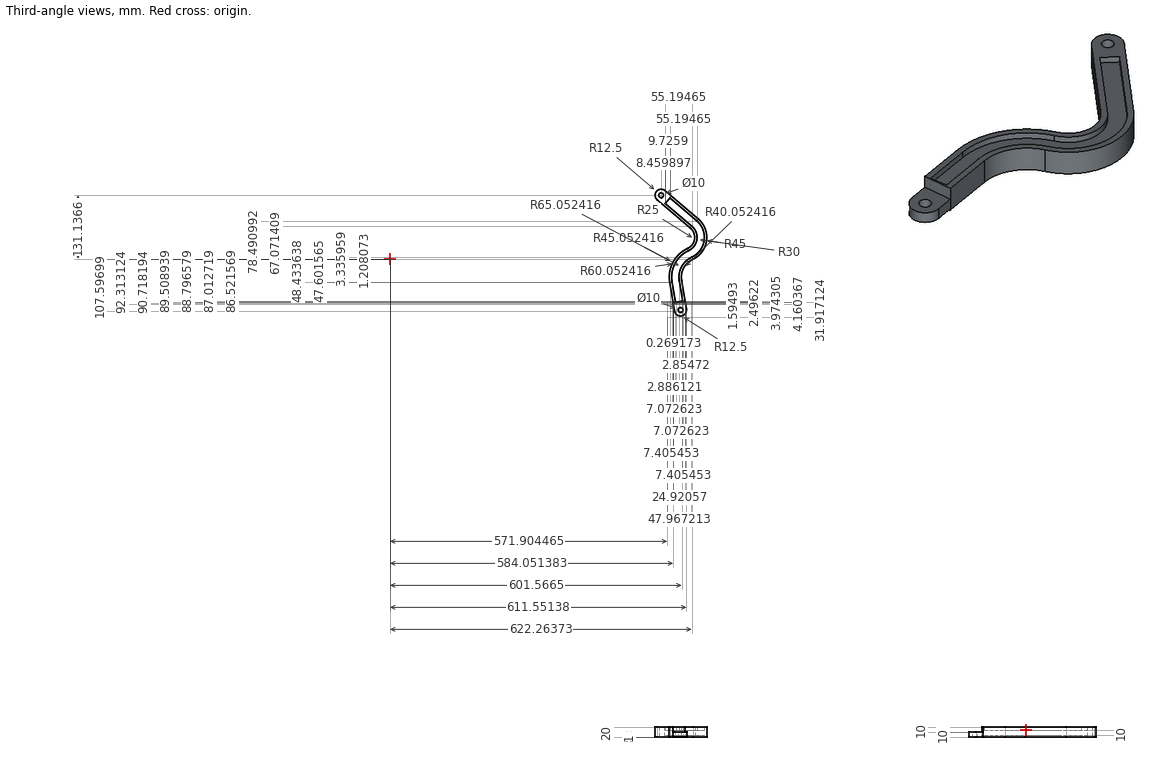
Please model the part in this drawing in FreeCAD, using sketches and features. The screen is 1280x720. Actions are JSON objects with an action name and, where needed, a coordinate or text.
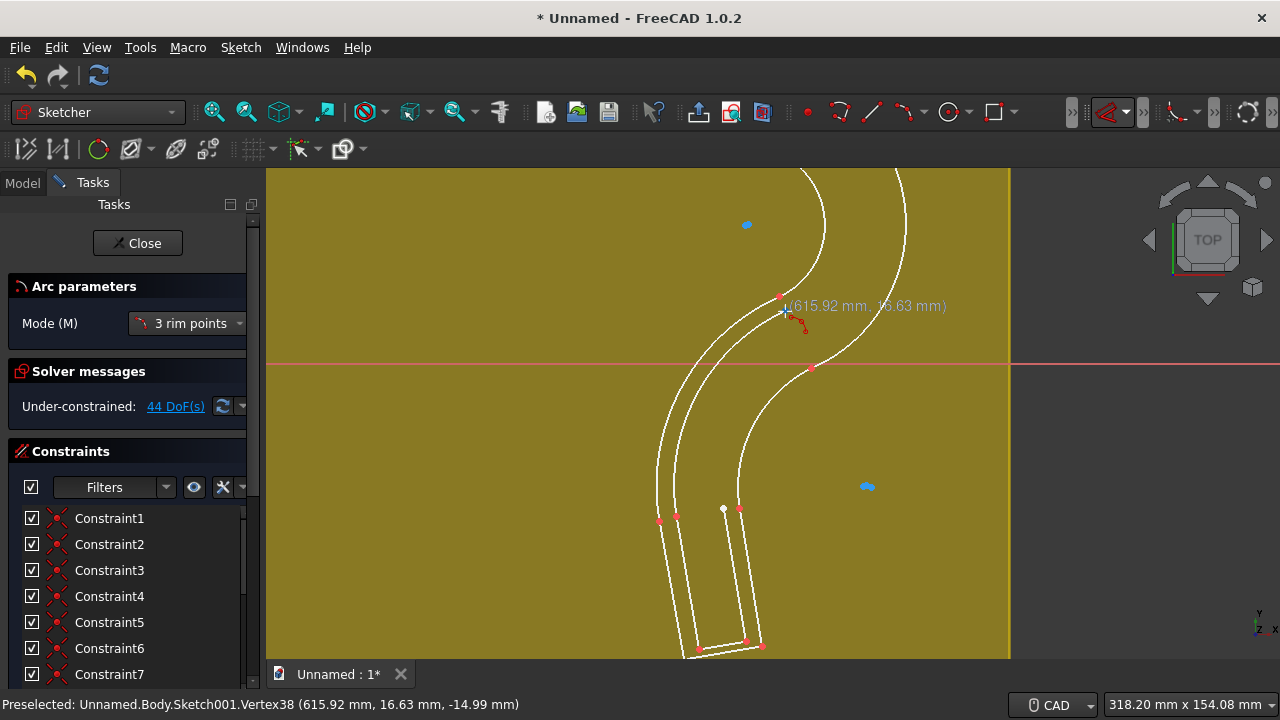
{"action": "scroll", "coordinate": [677, 517], "scroll_direction": "down", "scroll_amount": 4}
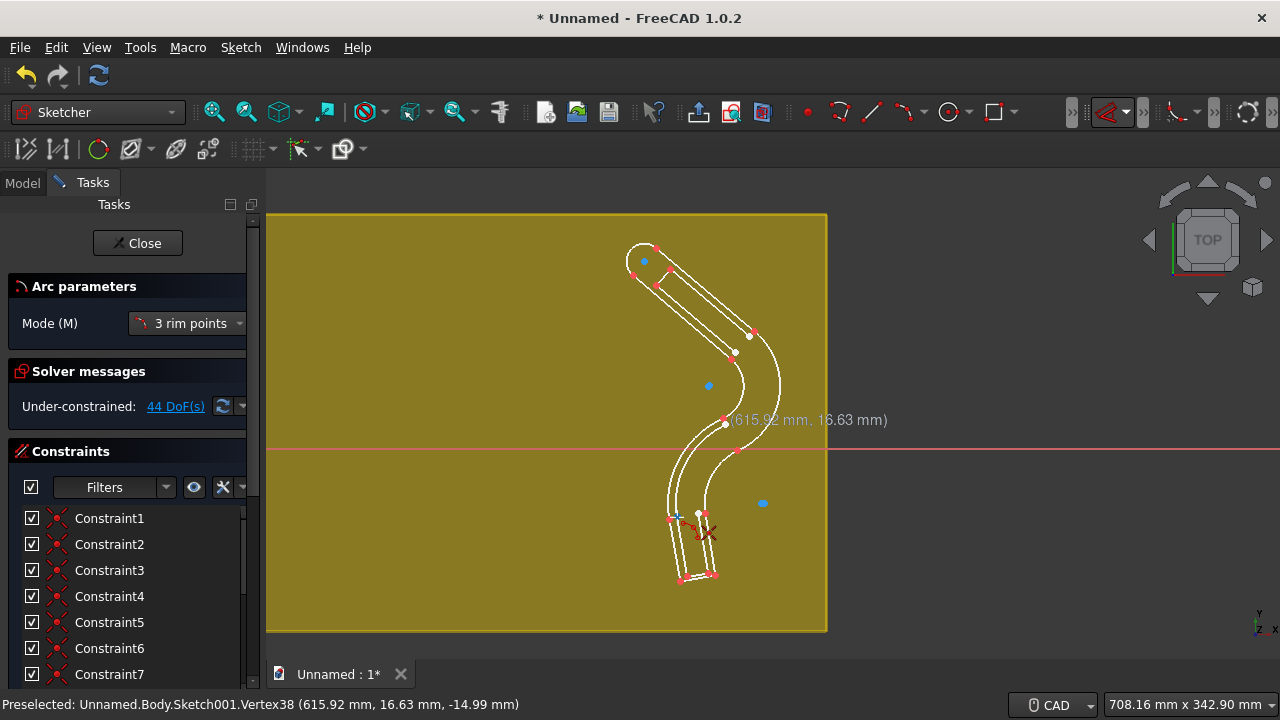
{"action": "scroll", "coordinate": [736, 353], "scroll_direction": "up", "scroll_amount": 4}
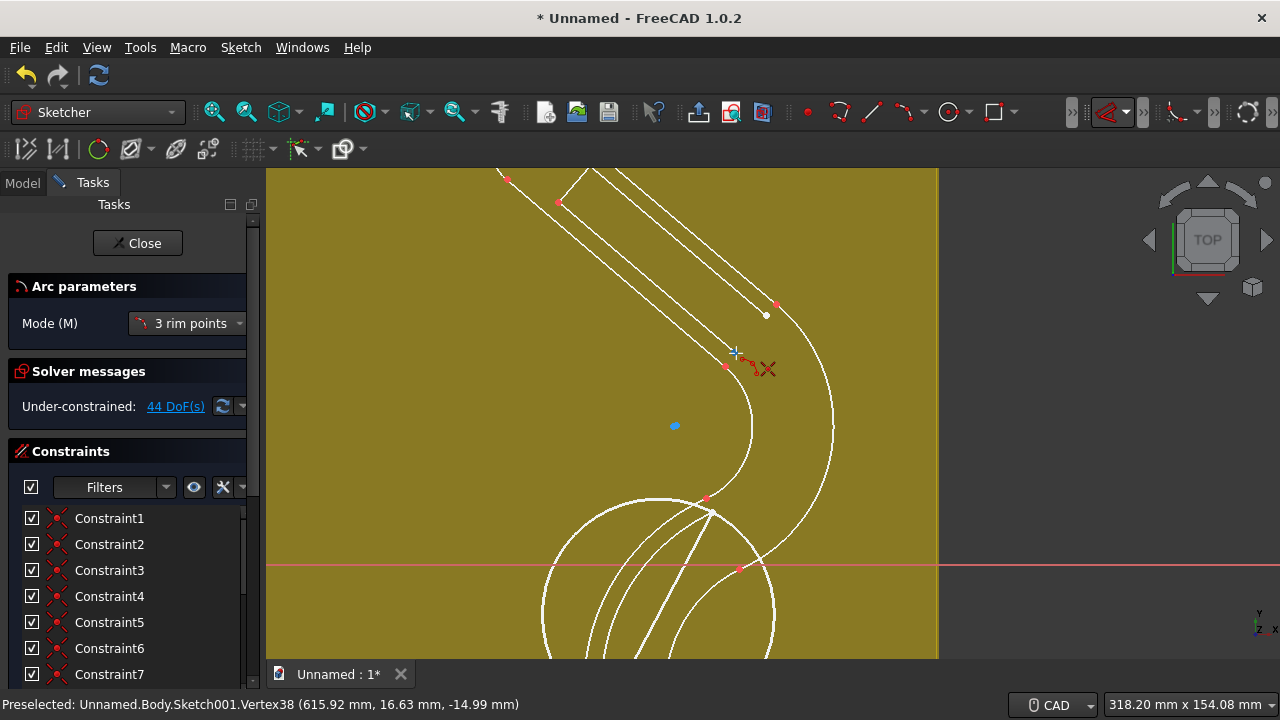
{"action": "left_click", "coordinate": [735, 352]}
{"action": "left_click", "coordinate": [768, 418]}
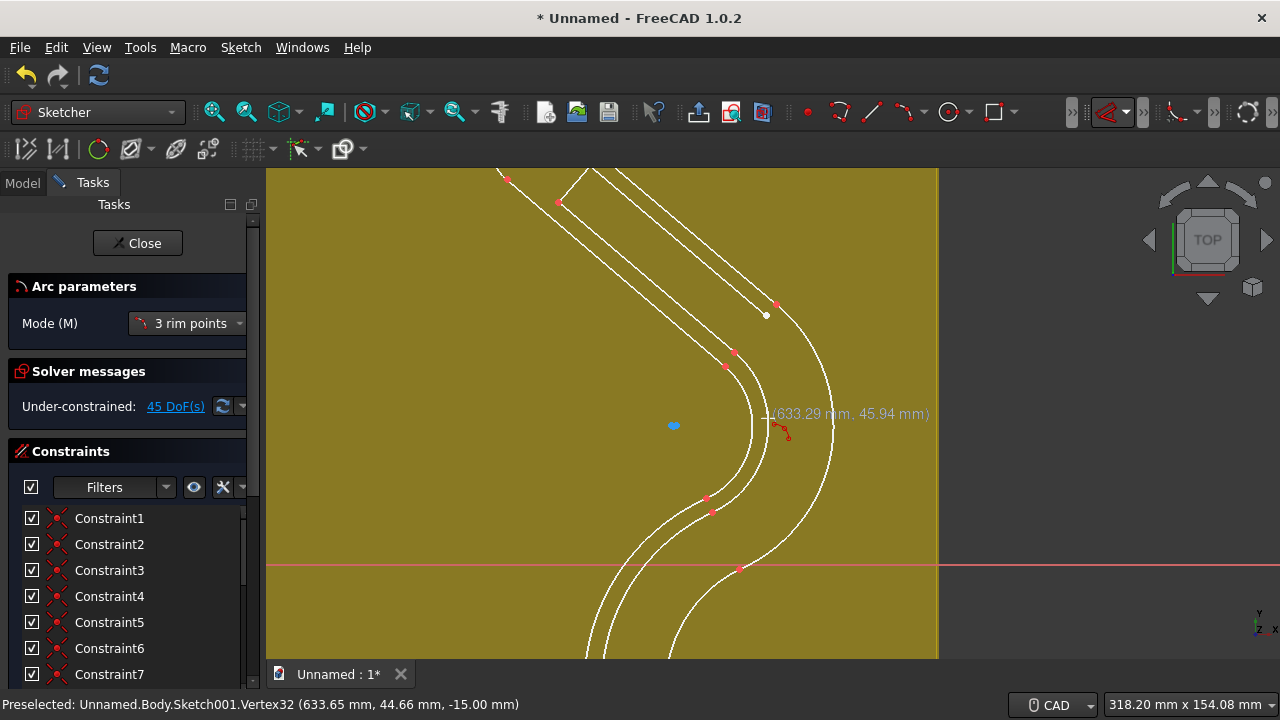
{"action": "left_click", "coordinate": [766, 316]}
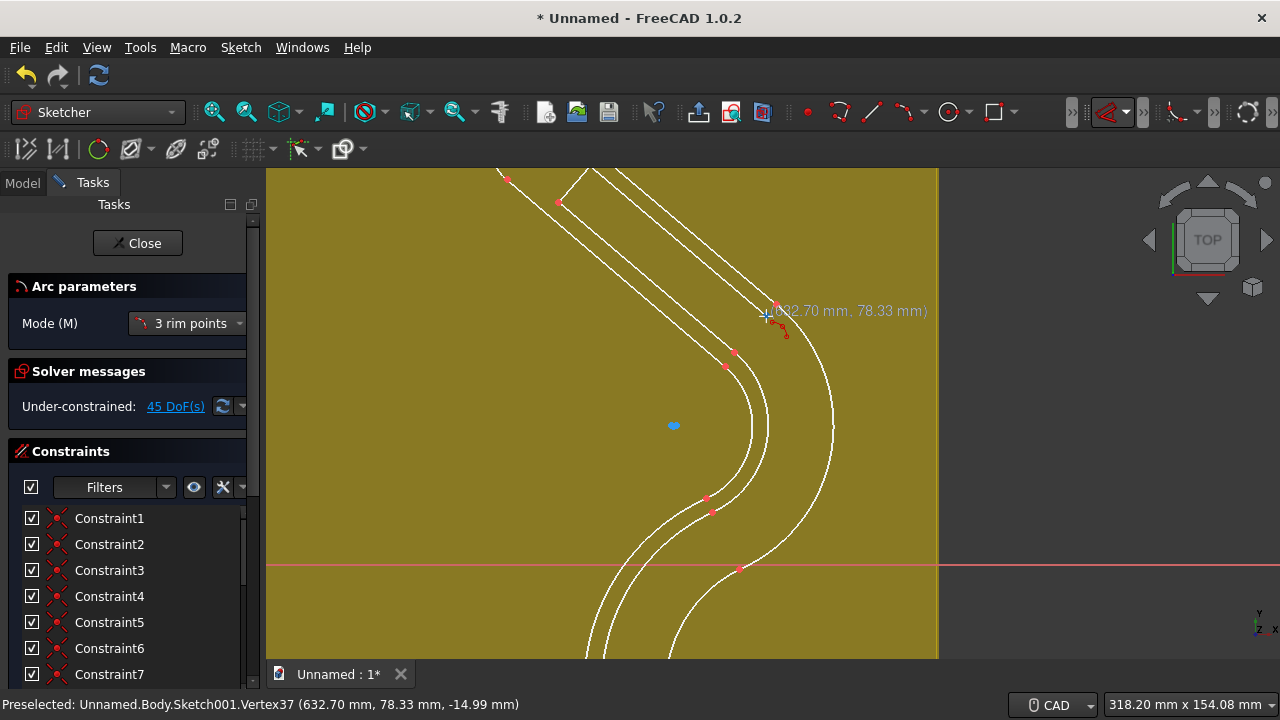
{"action": "scroll", "coordinate": [733, 555], "scroll_direction": "up", "scroll_amount": 3}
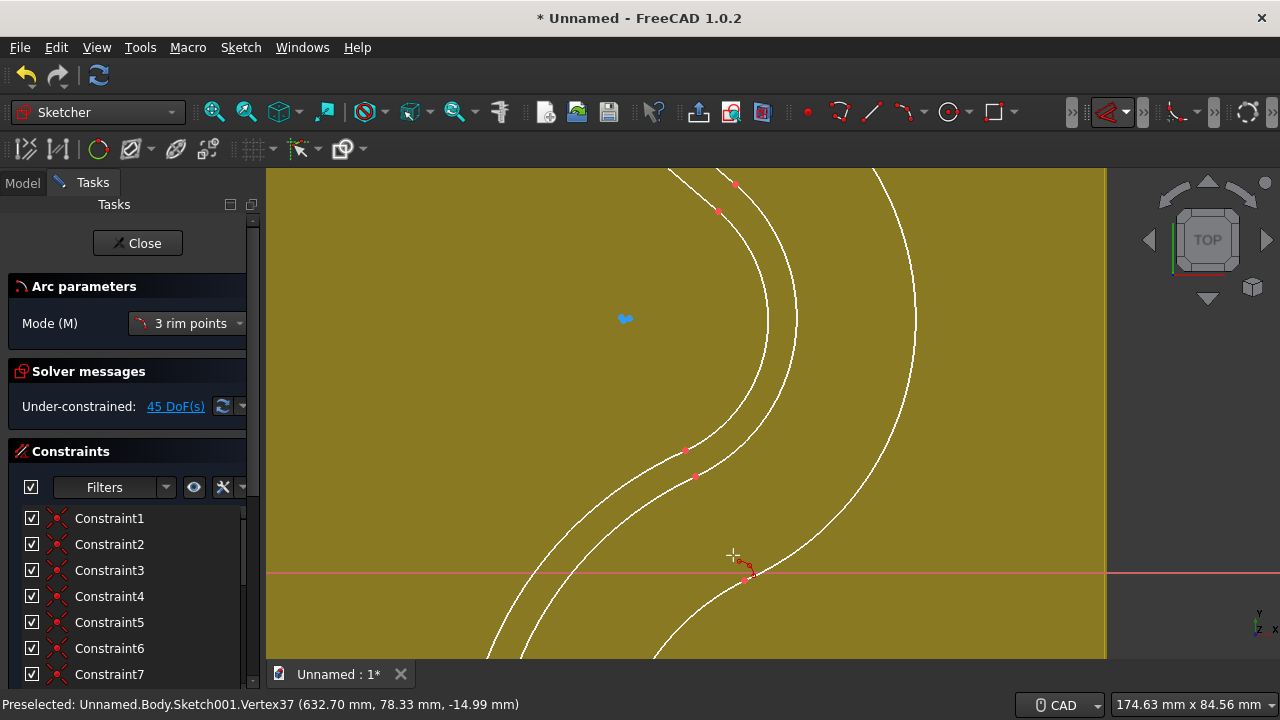
{"action": "left_click", "coordinate": [732, 554]}
{"action": "left_click", "coordinate": [884, 300]}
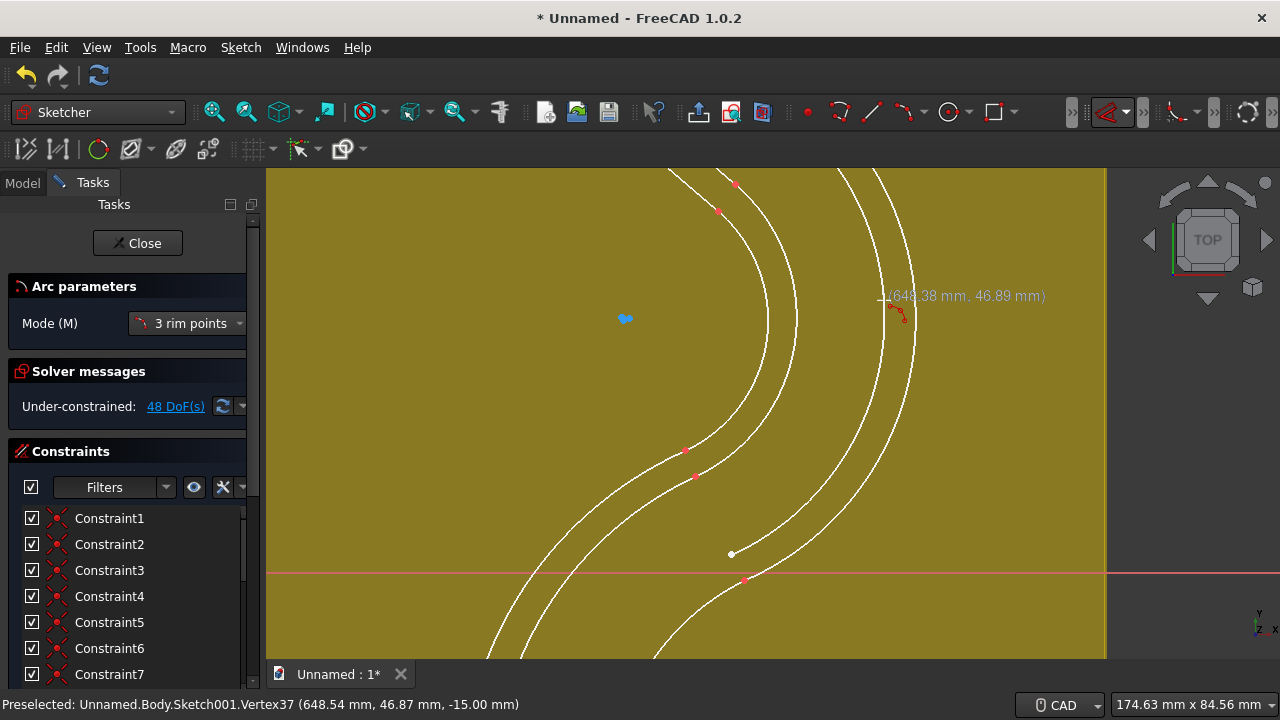
{"action": "left_click", "coordinate": [732, 555]}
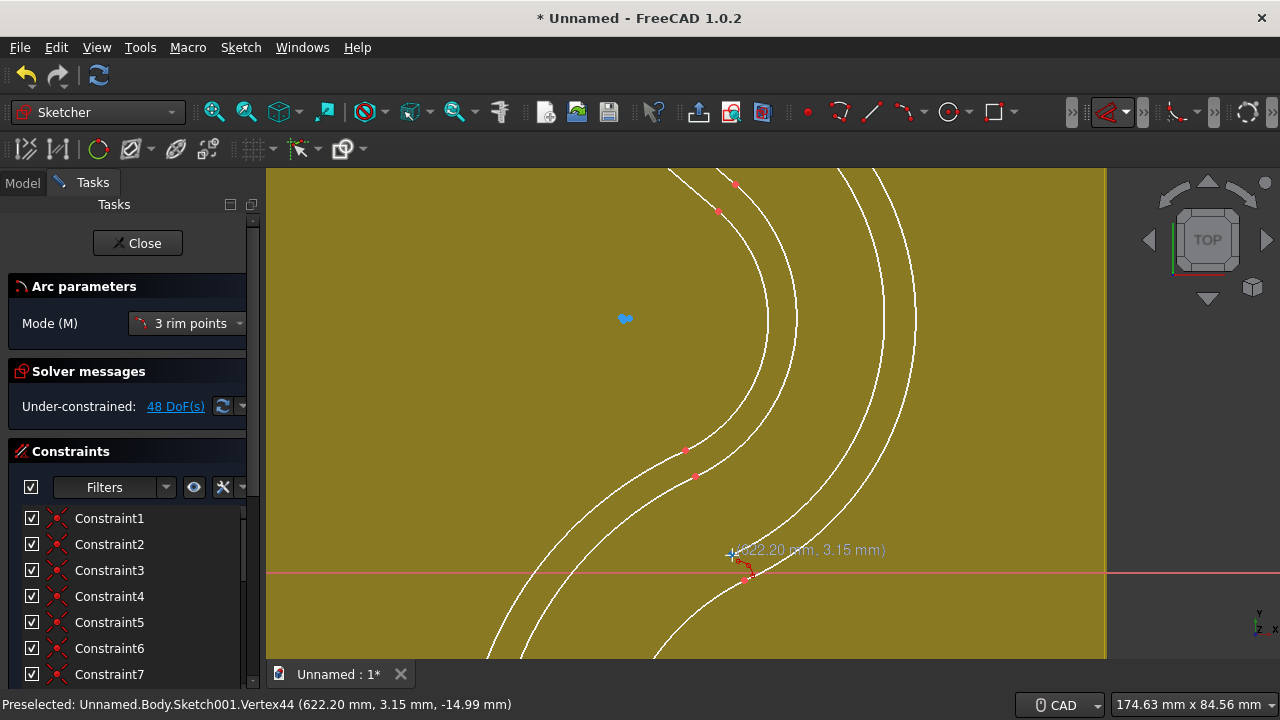
{"action": "scroll", "coordinate": [735, 407], "scroll_direction": "down", "scroll_amount": 7}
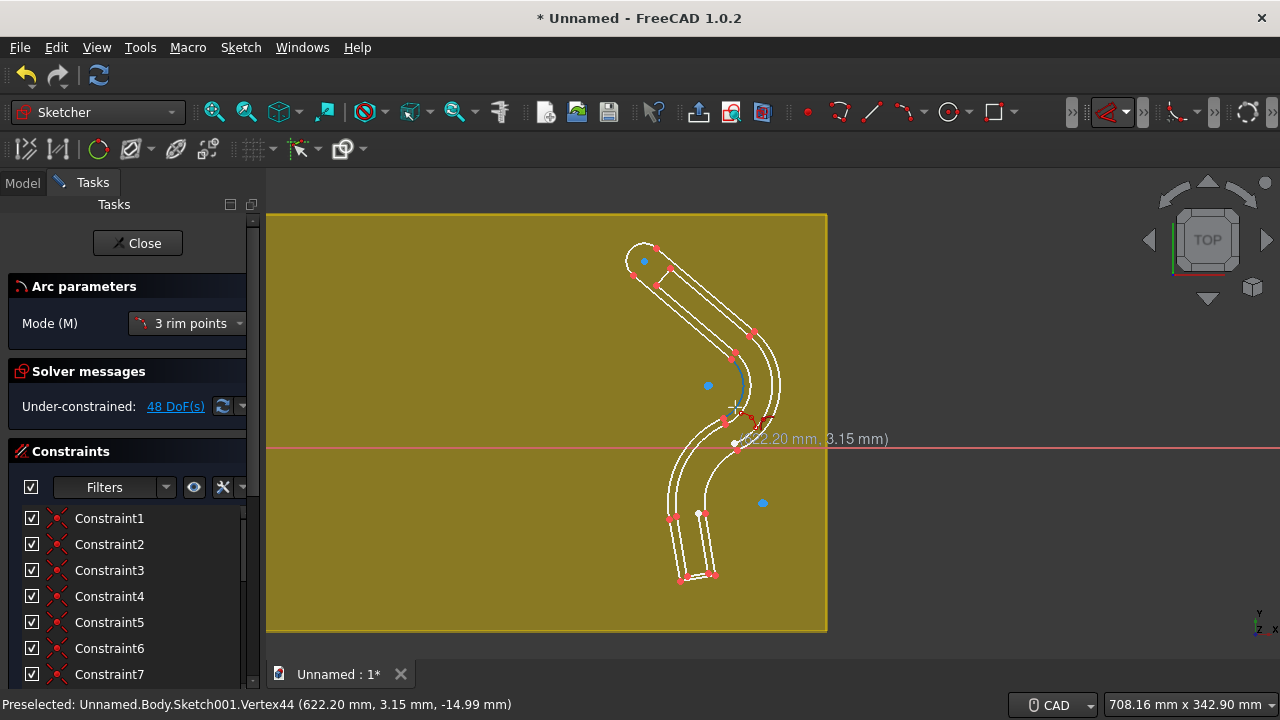
{"action": "scroll", "coordinate": [698, 513], "scroll_direction": "up", "scroll_amount": 4}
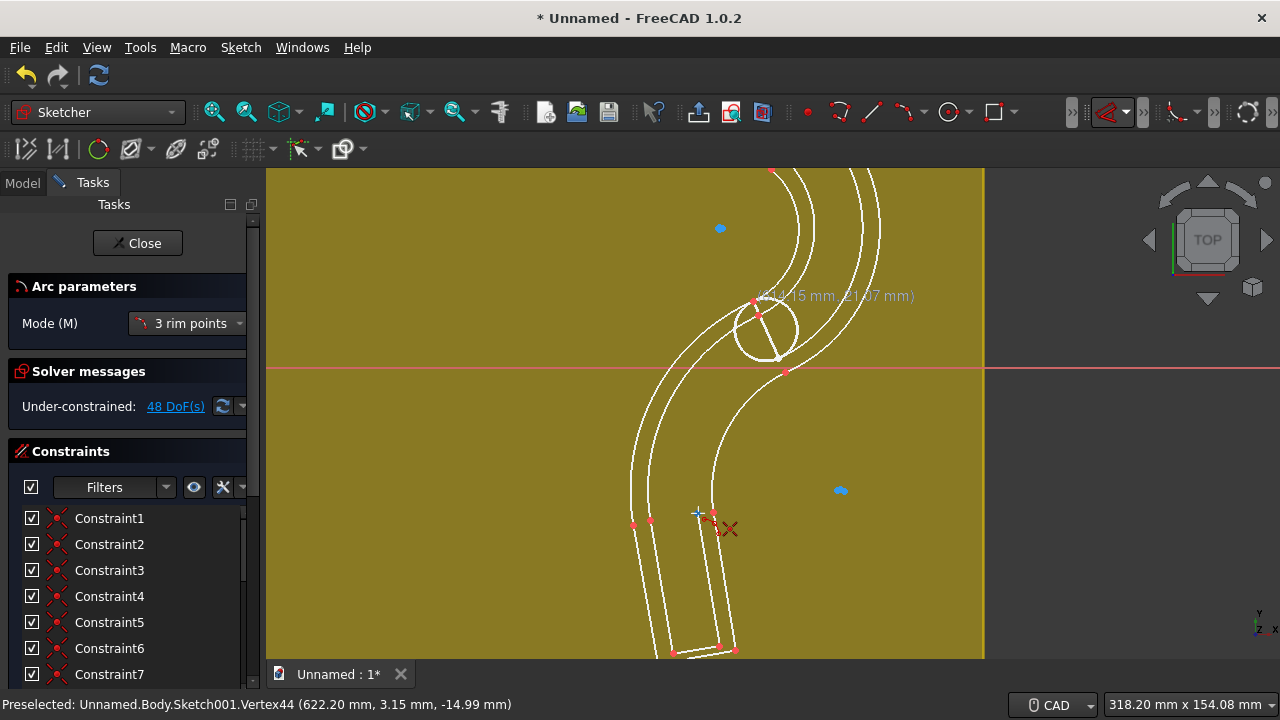
{"action": "left_click", "coordinate": [698, 513]}
{"action": "left_click", "coordinate": [712, 421]}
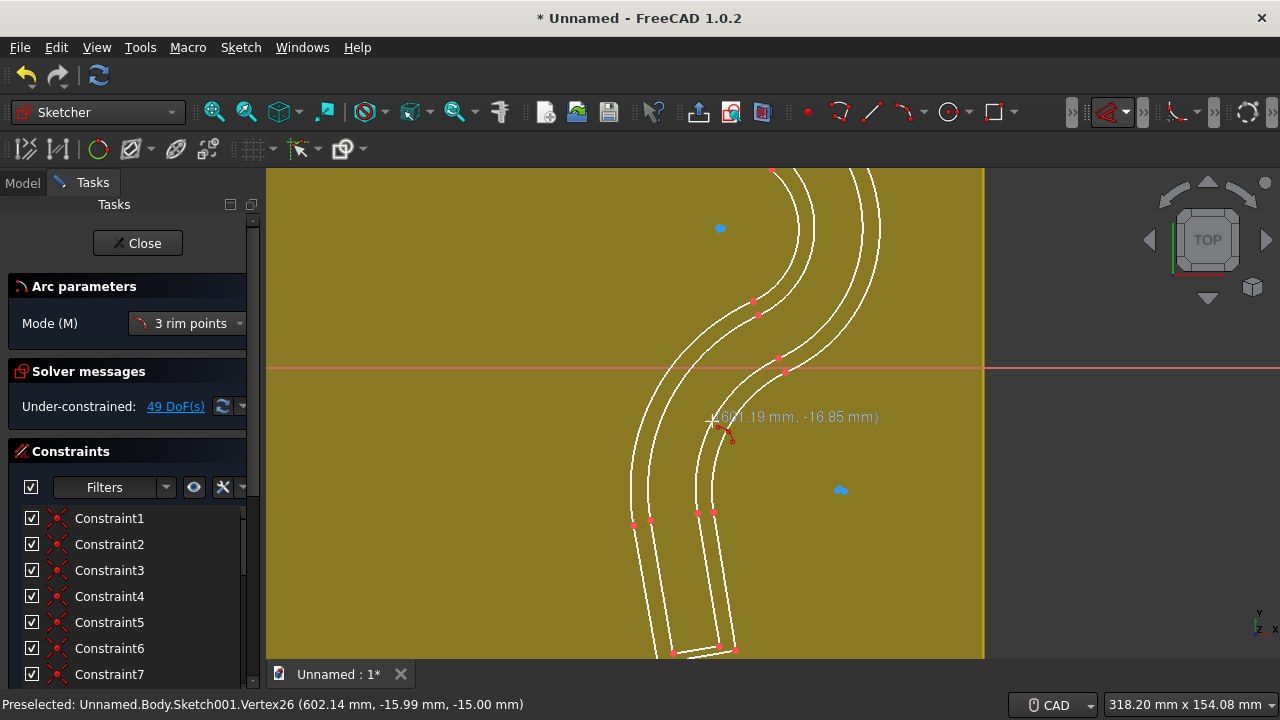
{"action": "left_click", "coordinate": [950, 112]}